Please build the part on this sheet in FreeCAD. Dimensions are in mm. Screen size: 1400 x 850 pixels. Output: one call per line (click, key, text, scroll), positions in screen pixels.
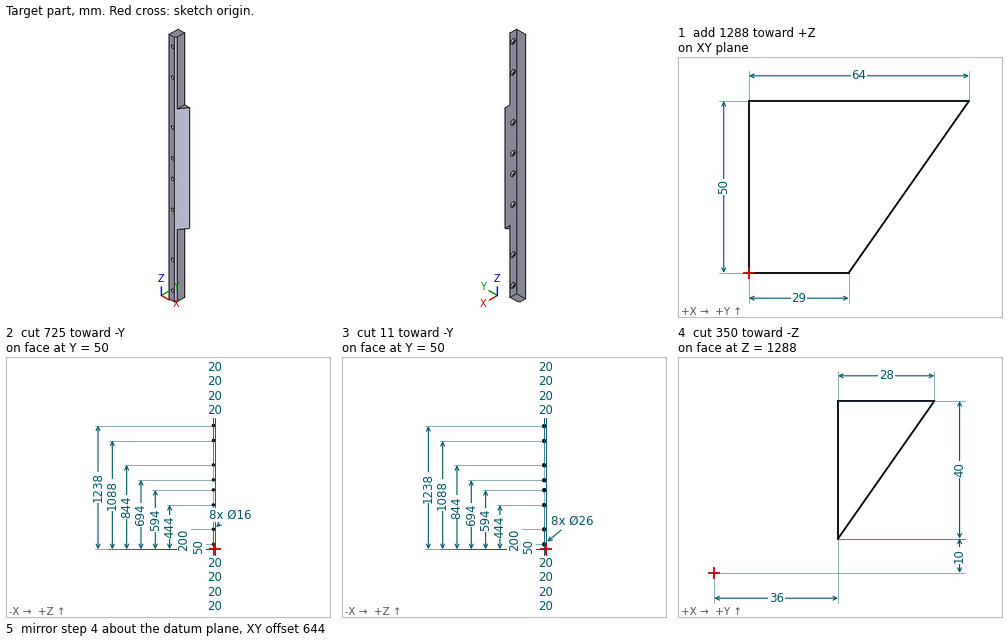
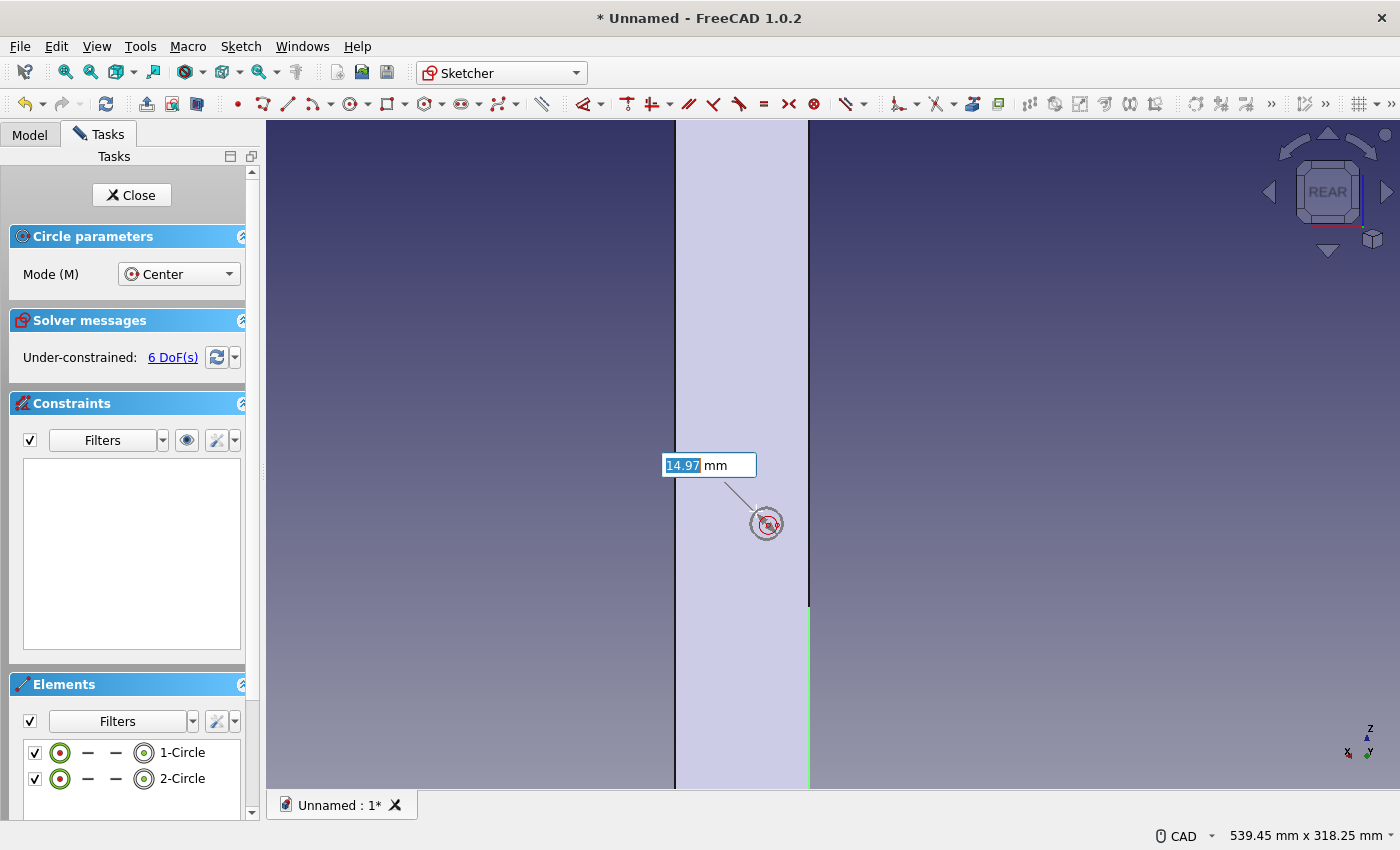
click(755, 510)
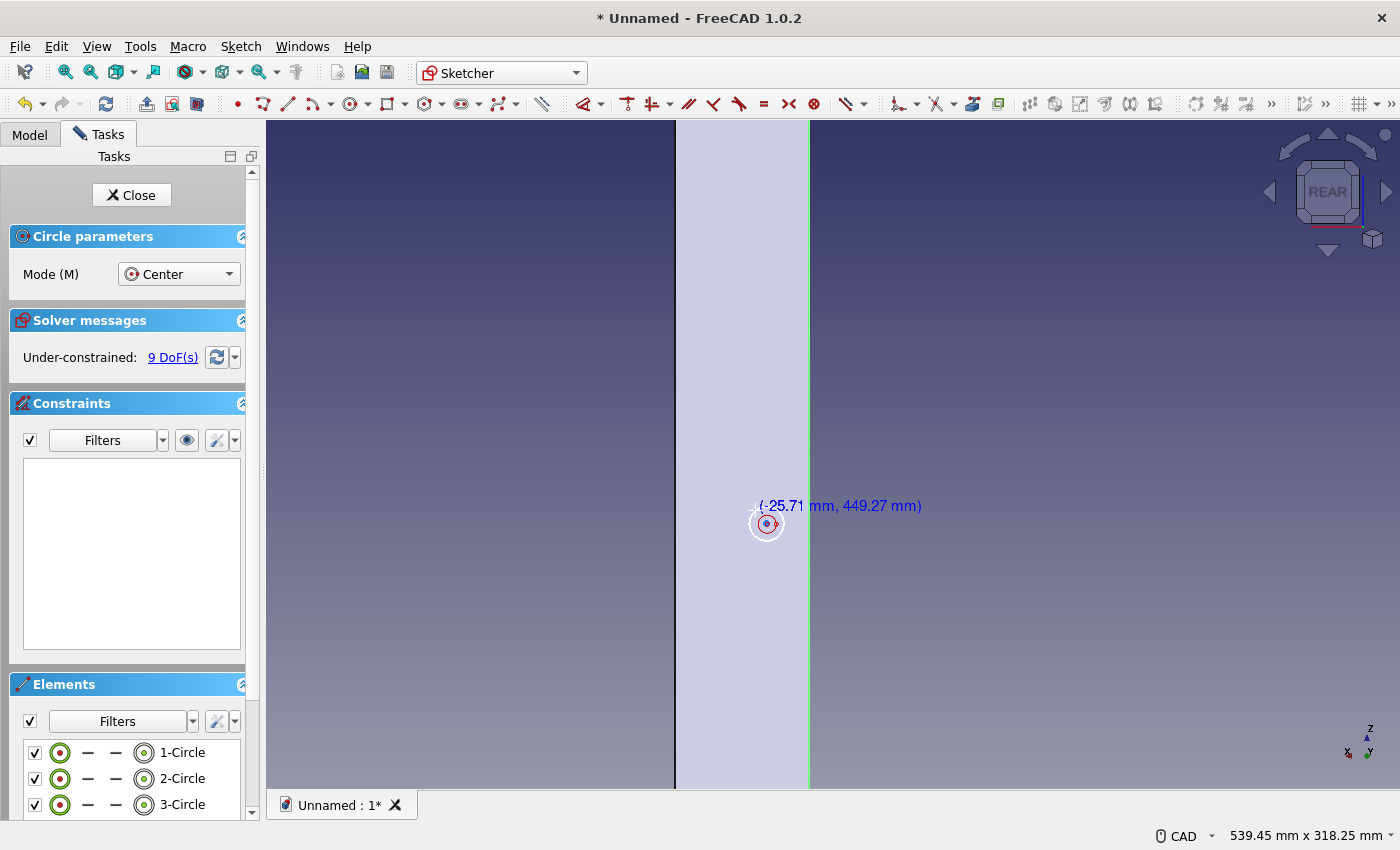
scroll(767, 207, up, 2)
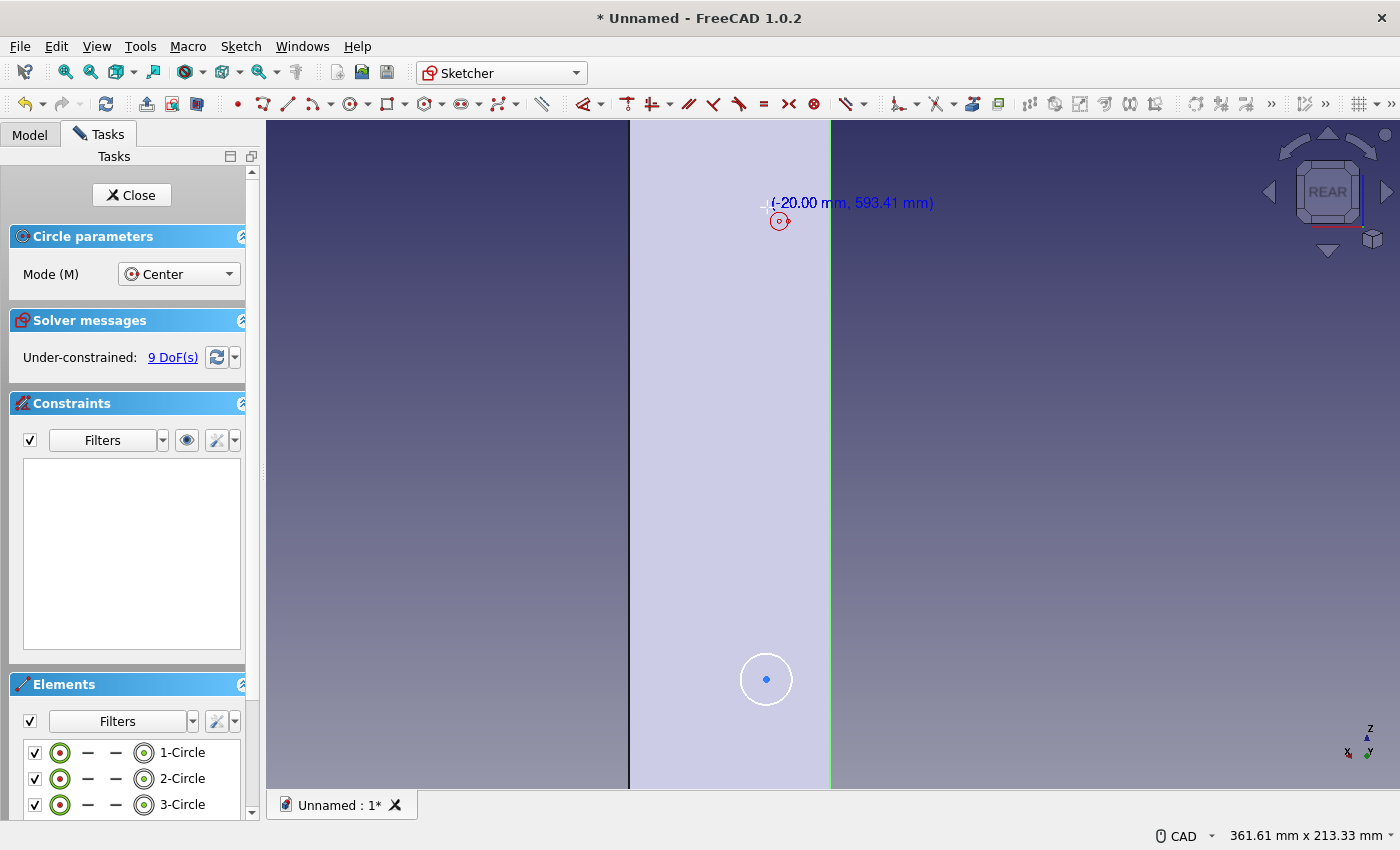
scroll(762, 497, down, 11)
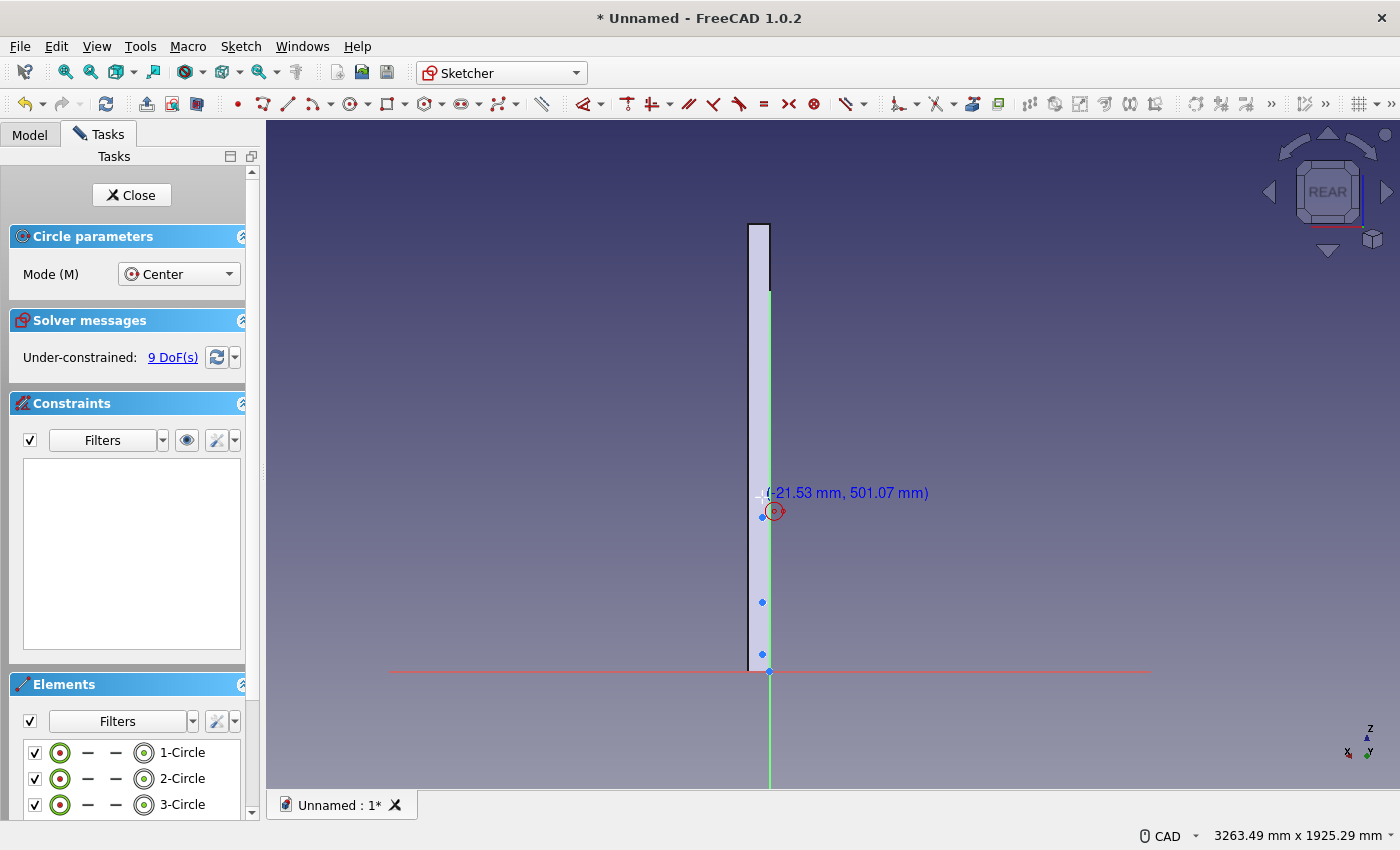
scroll(763, 465, up, 5)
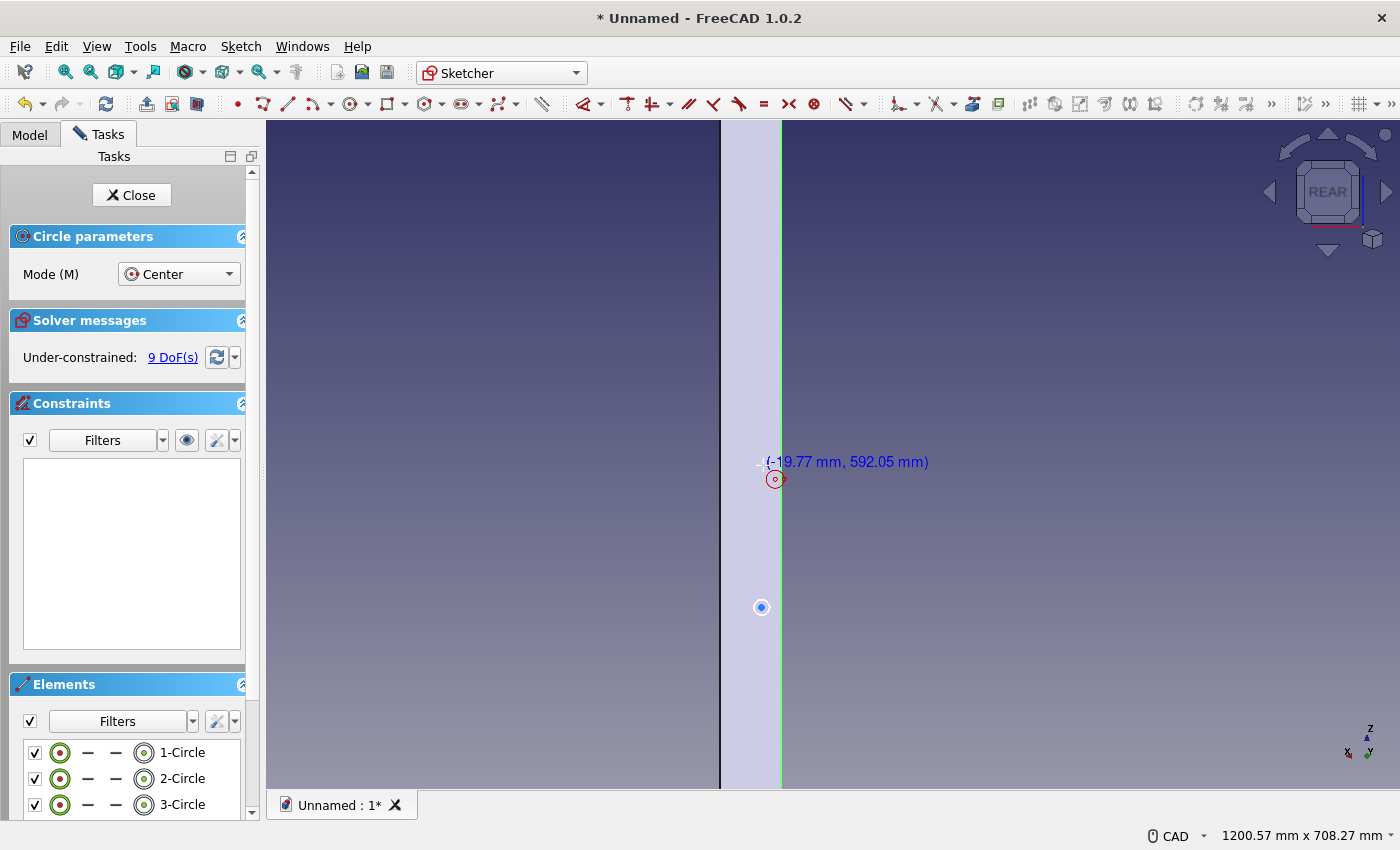
click(762, 465)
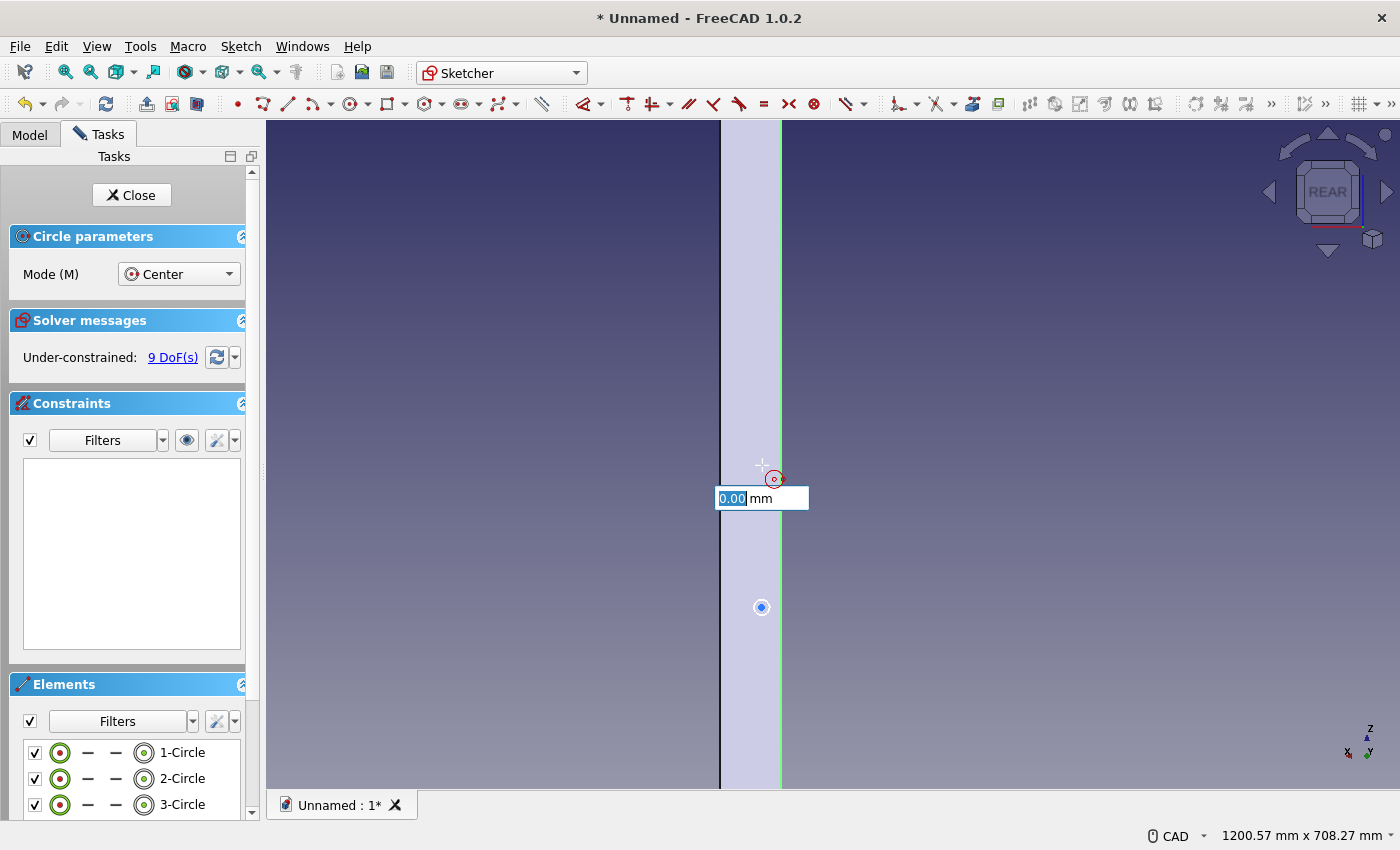
scroll(757, 460, up, 4)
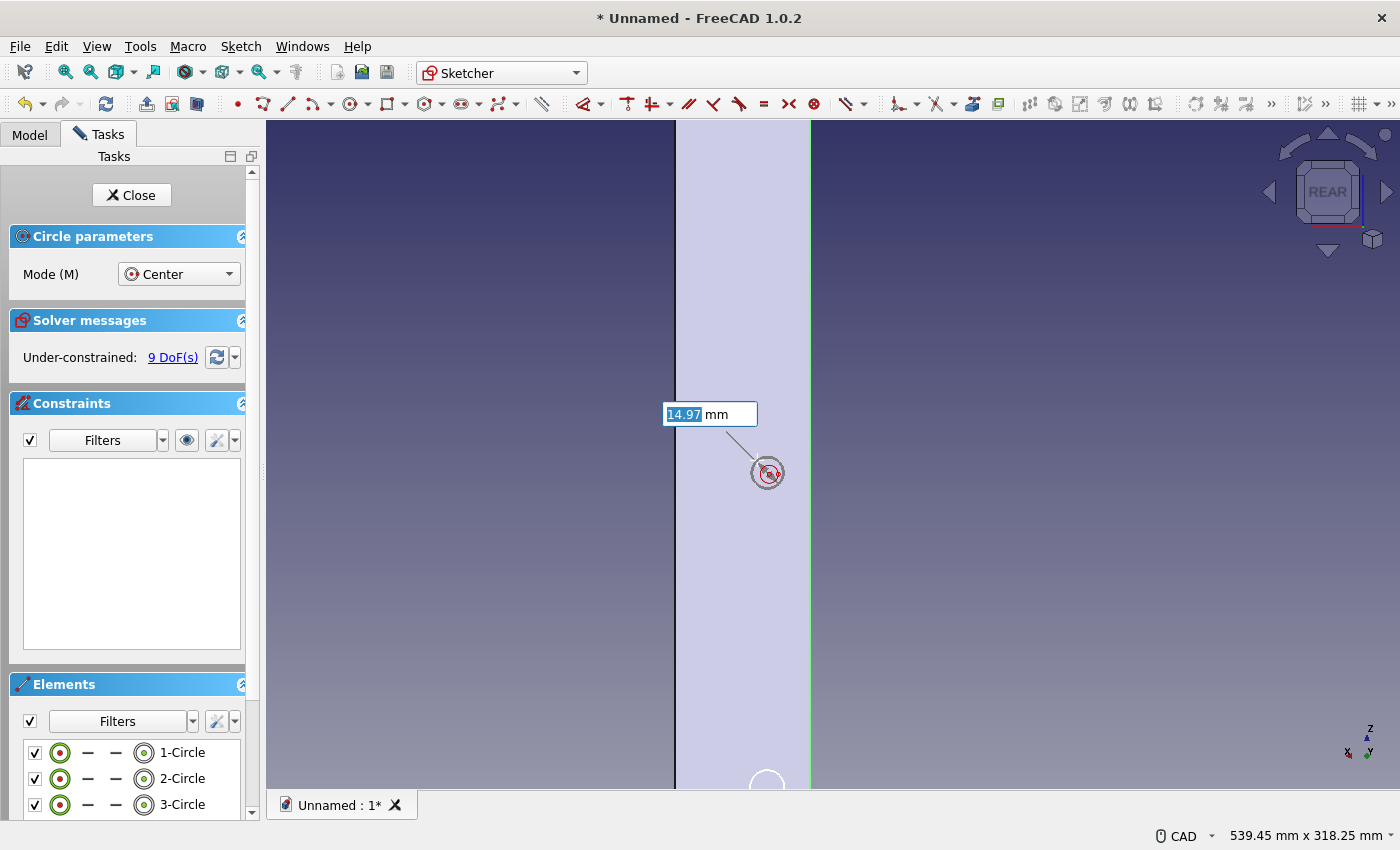
click(756, 459)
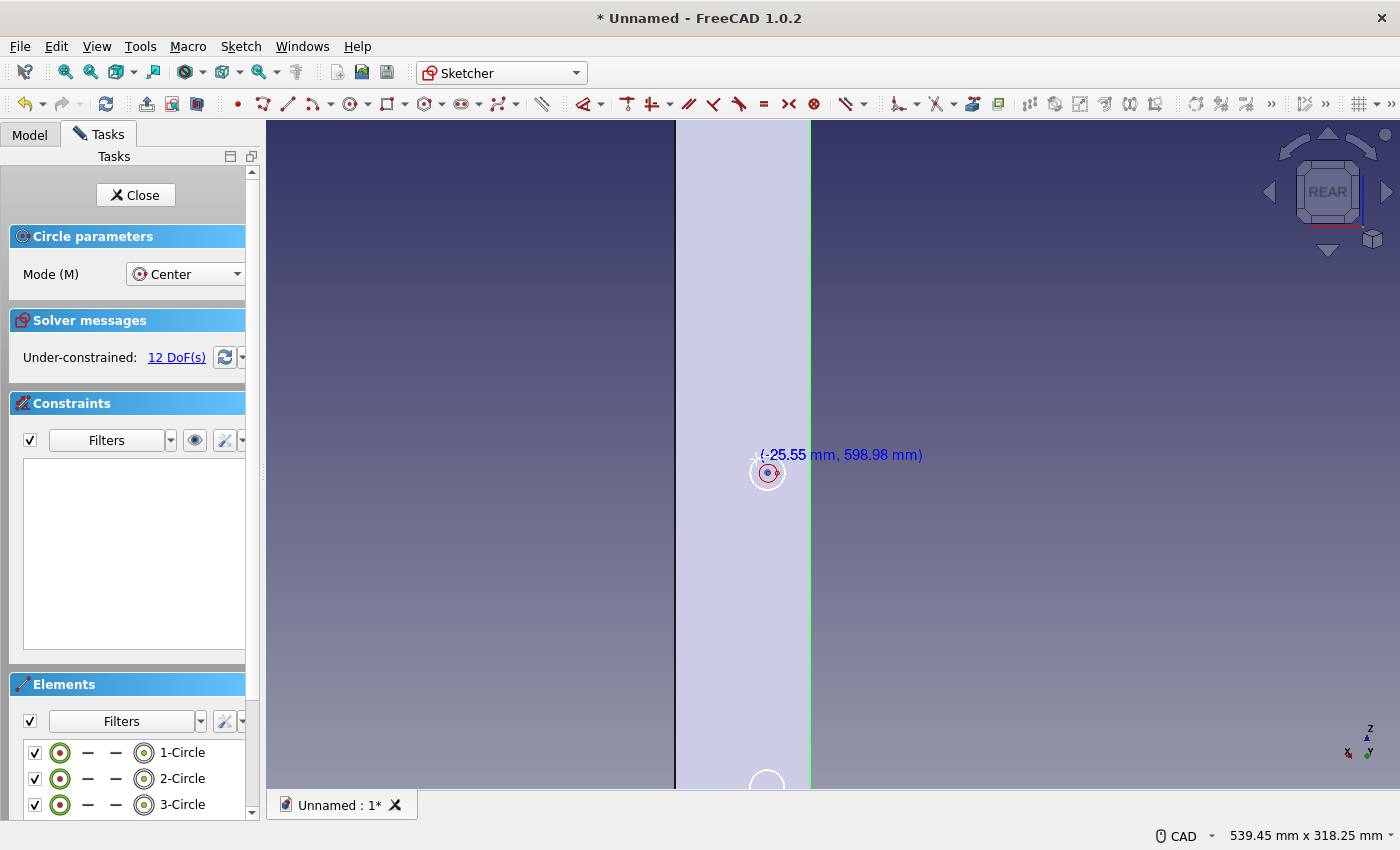
scroll(768, 260, up, 2)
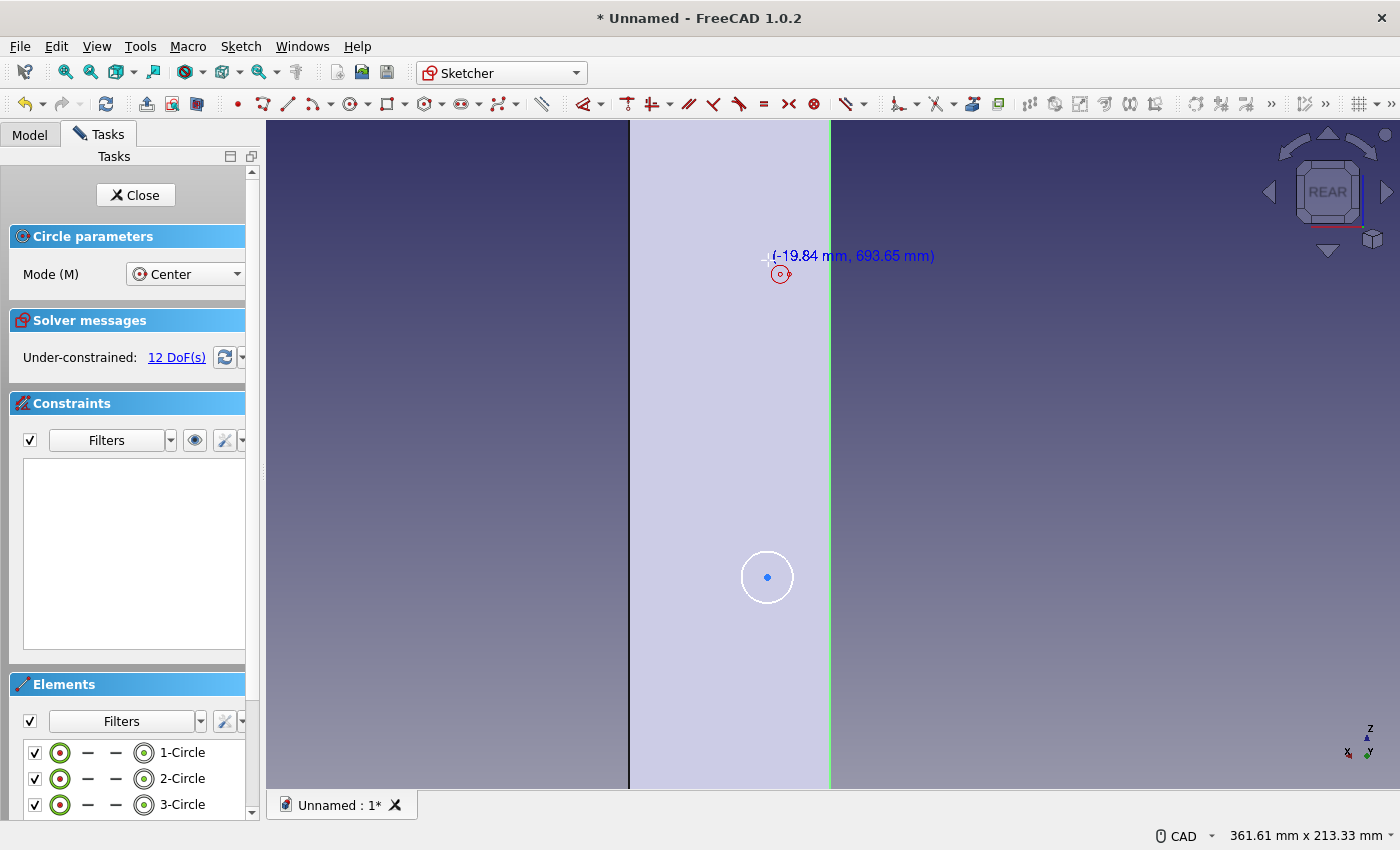
scroll(762, 451, down, 11)